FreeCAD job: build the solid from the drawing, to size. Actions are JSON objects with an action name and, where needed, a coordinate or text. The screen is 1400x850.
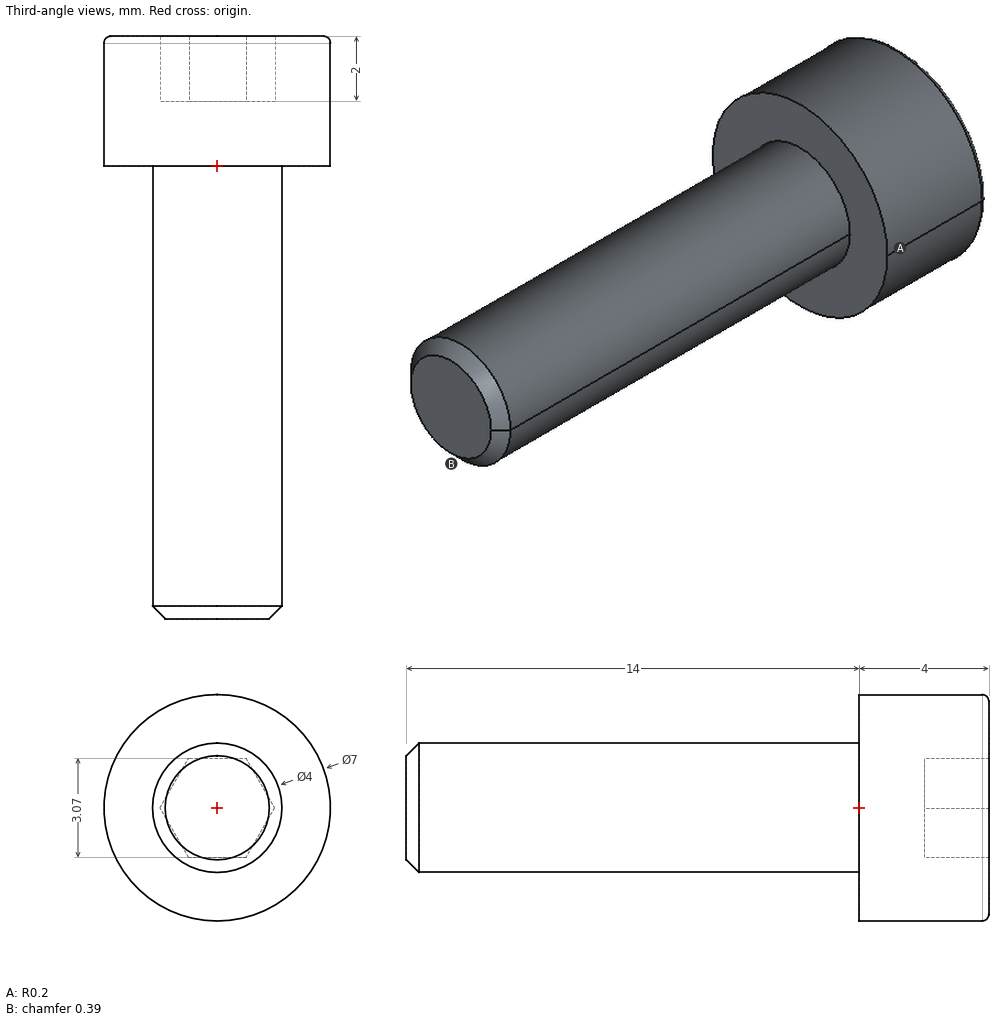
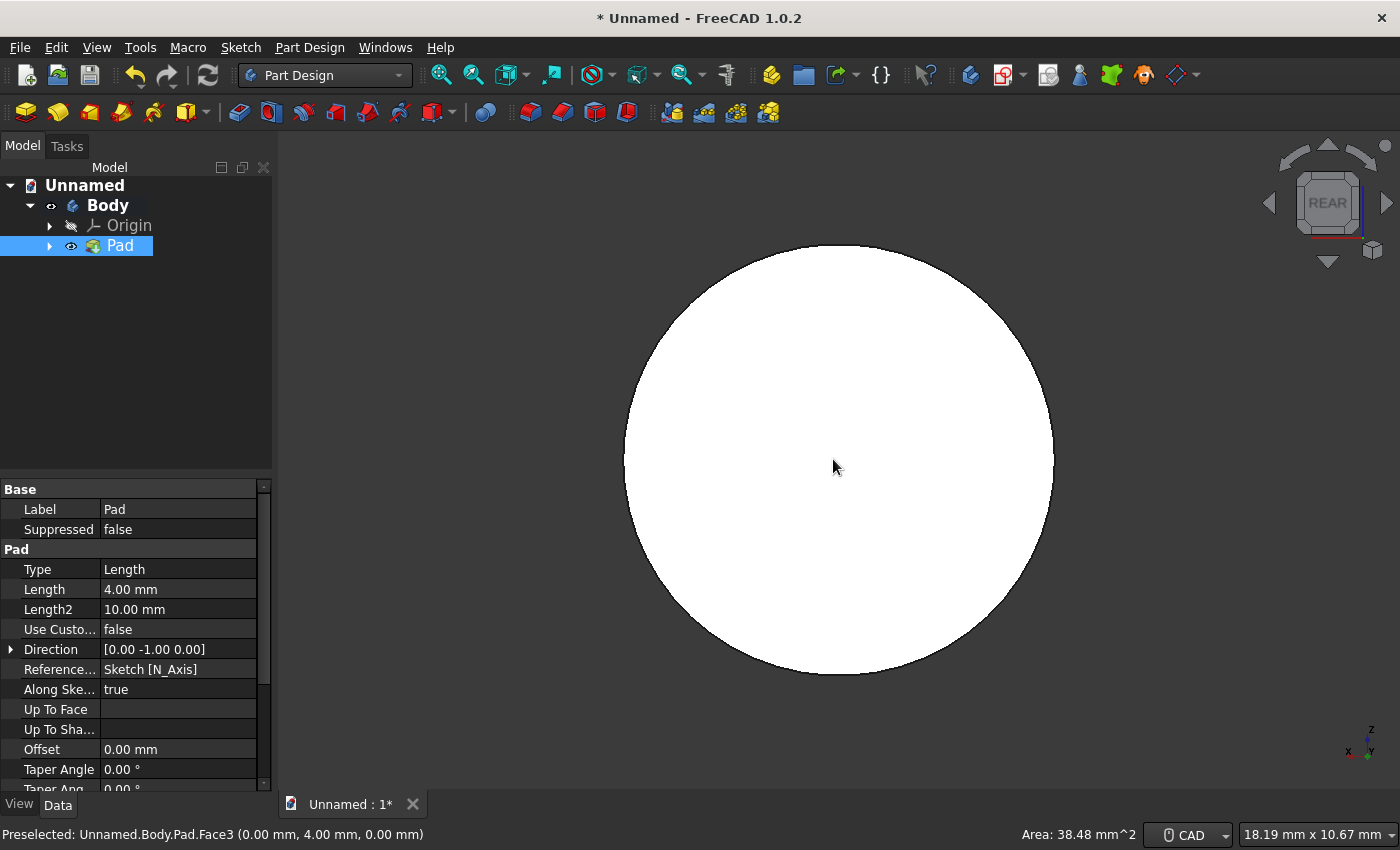
{"action": "left_click", "coordinate": [1004, 76]}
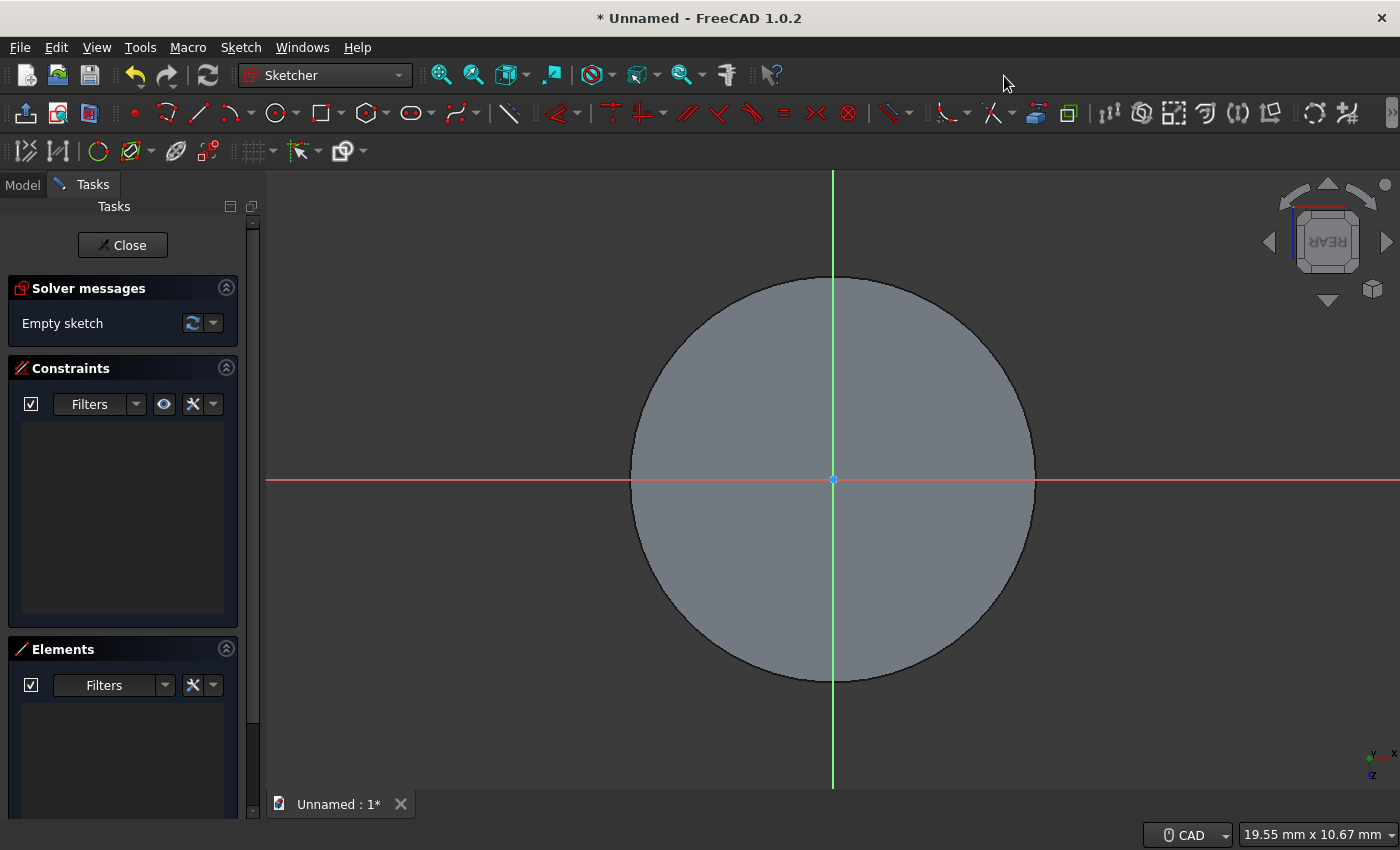
{"action": "scroll", "coordinate": [889, 480], "scroll_direction": "up", "scroll_amount": 4}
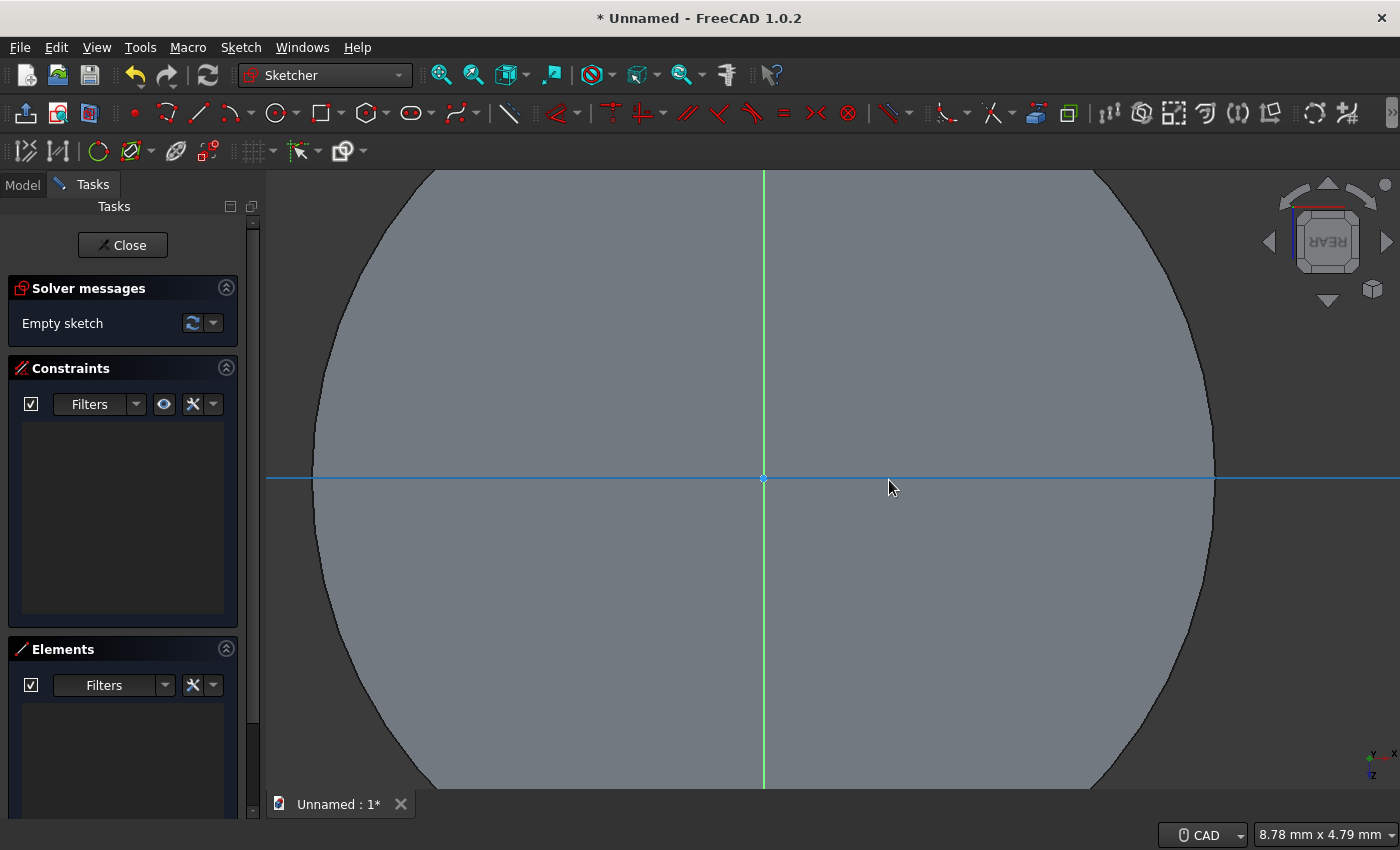
{"action": "left_click", "coordinate": [366, 114]}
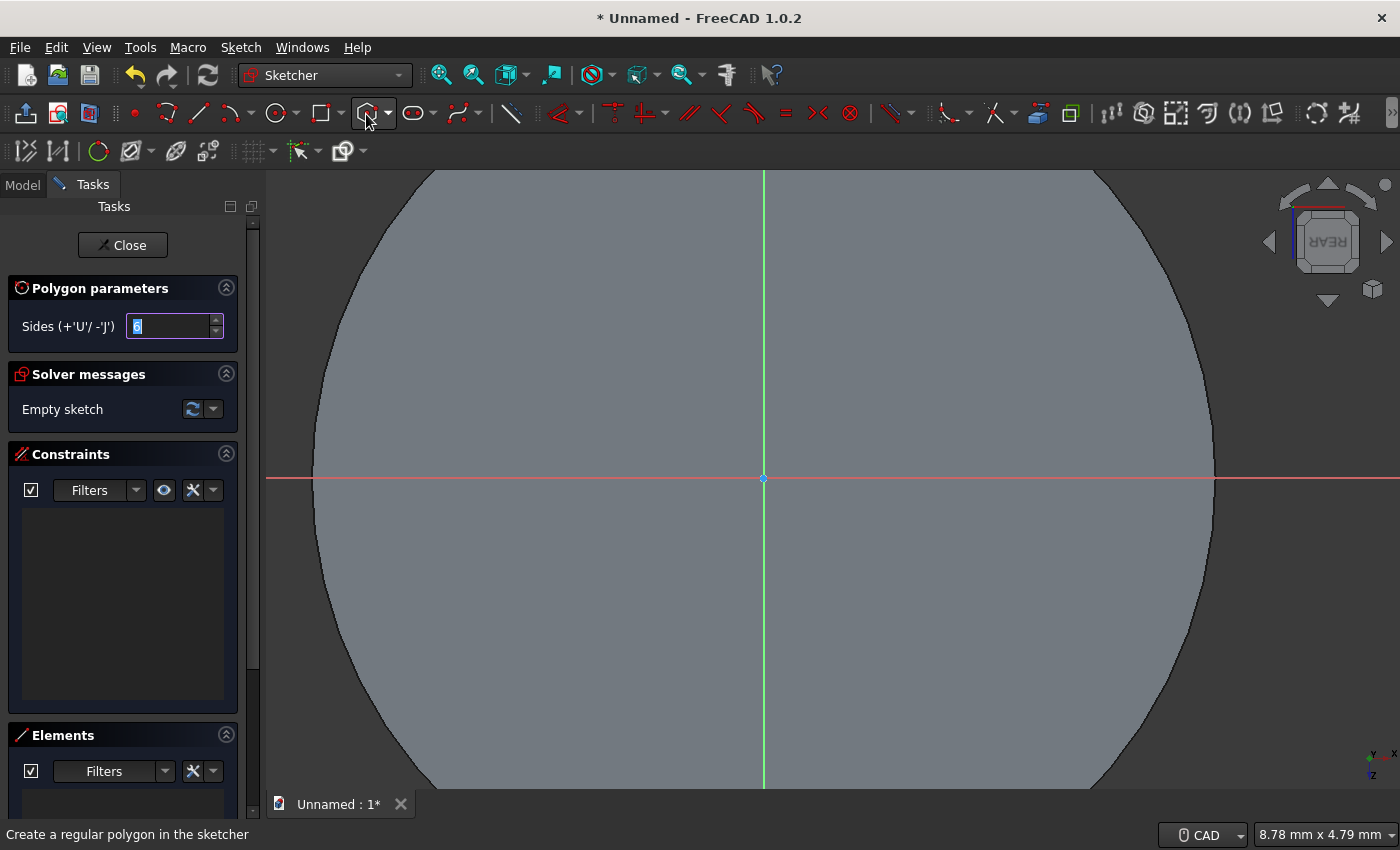
{"action": "left_click", "coordinate": [764, 478]}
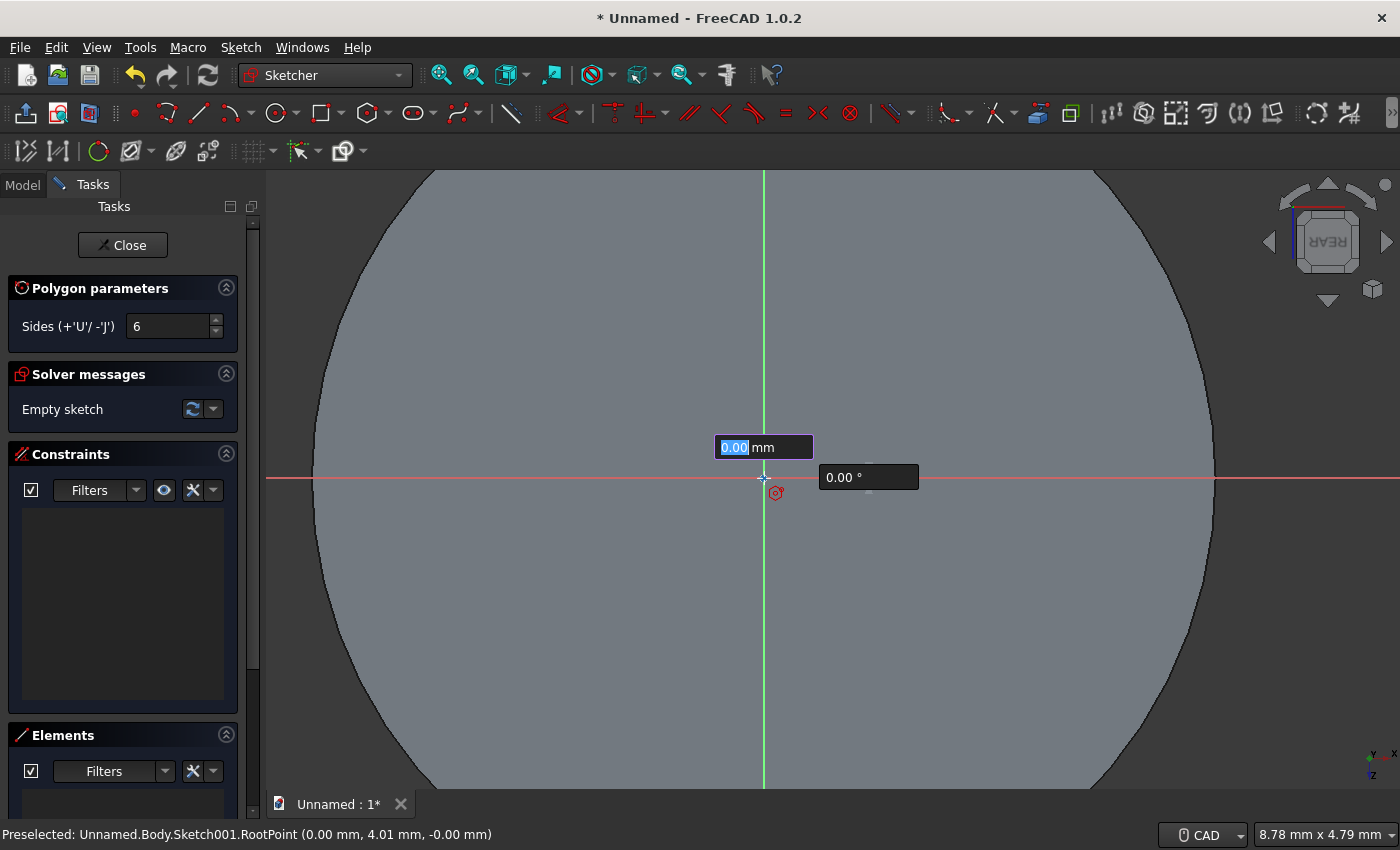
{"action": "left_click", "coordinate": [993, 478]}
{"action": "right_click", "coordinate": [993, 478]}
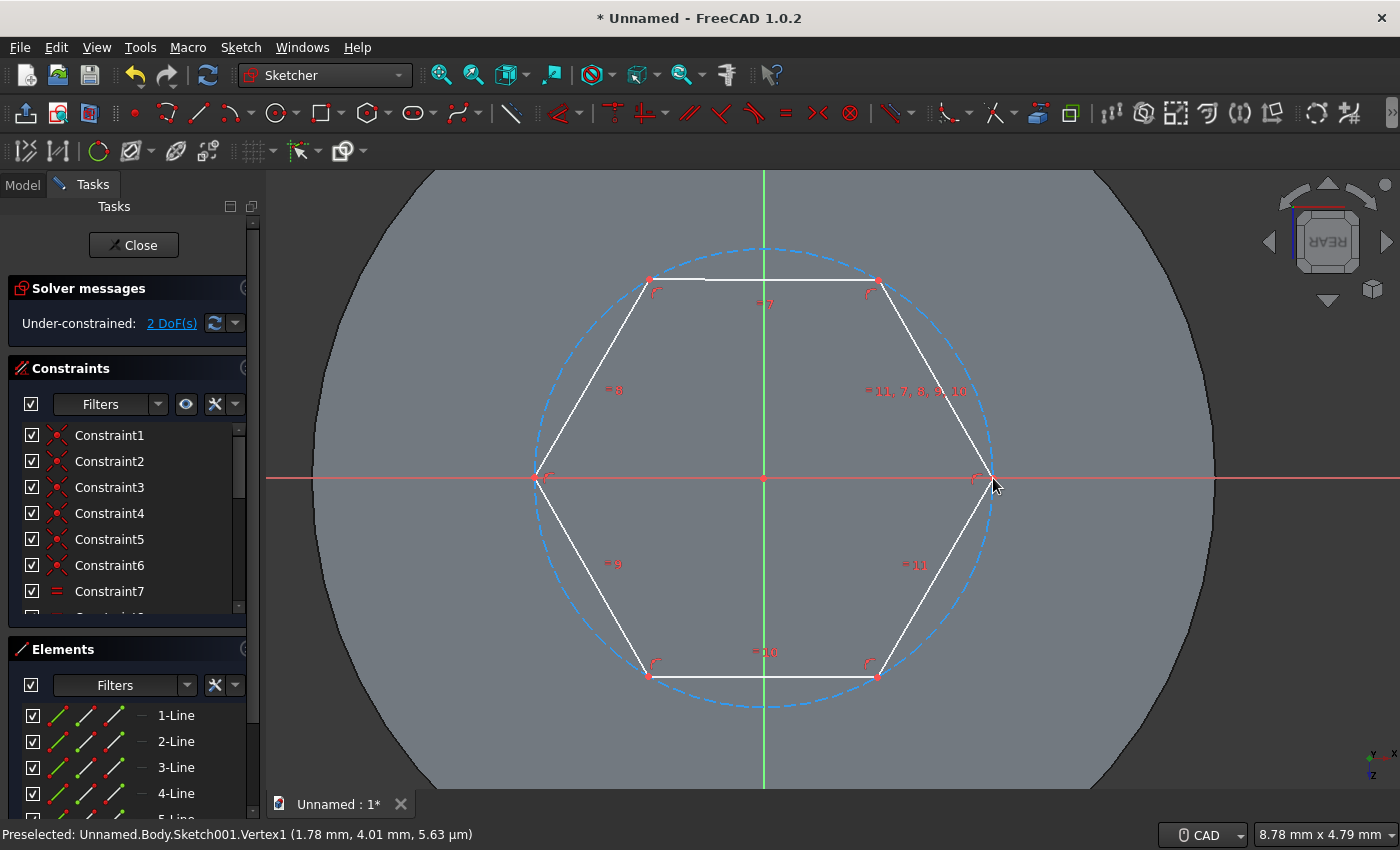
{"action": "left_click", "coordinate": [810, 280]}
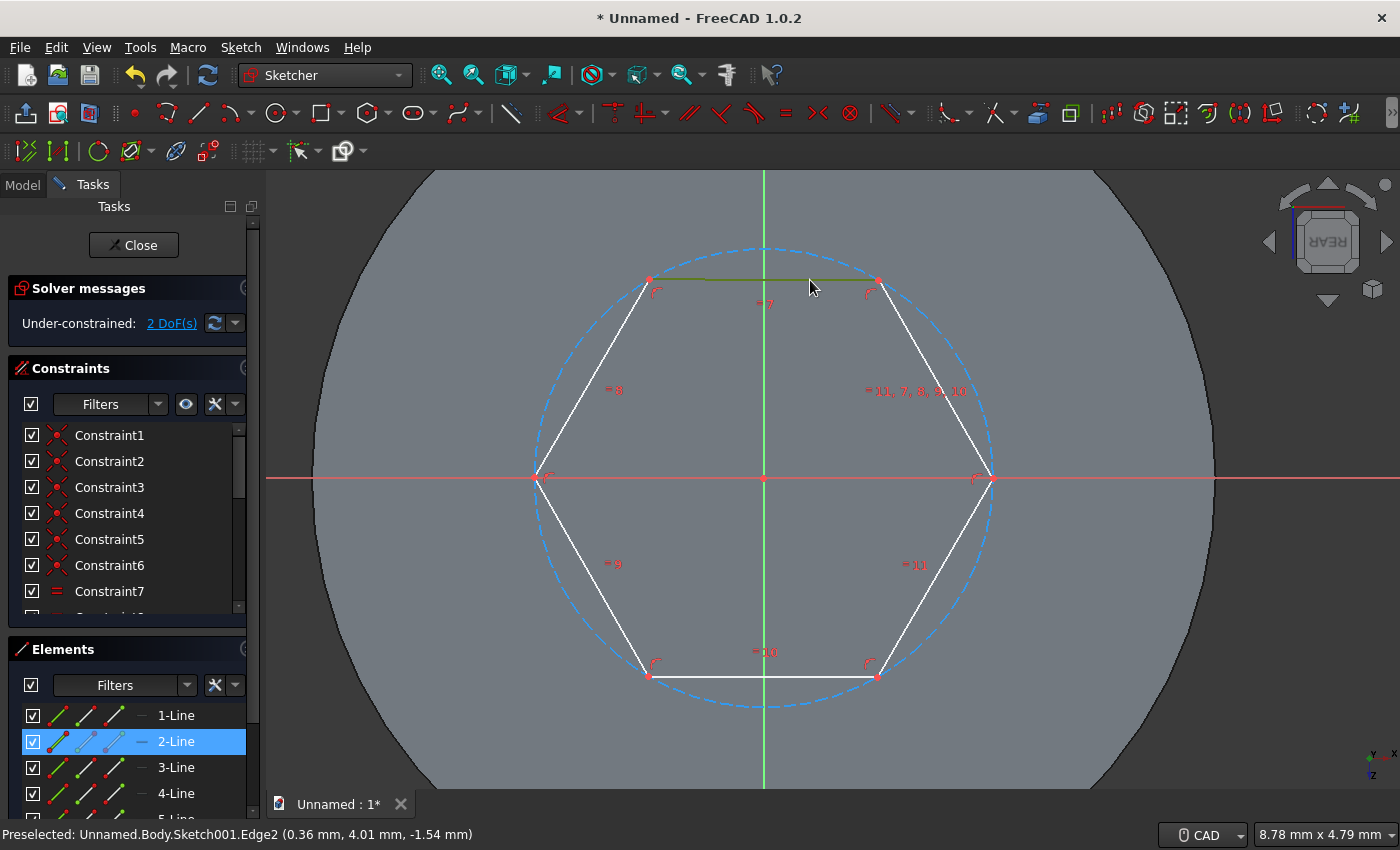
{"action": "left_click", "coordinate": [668, 114]}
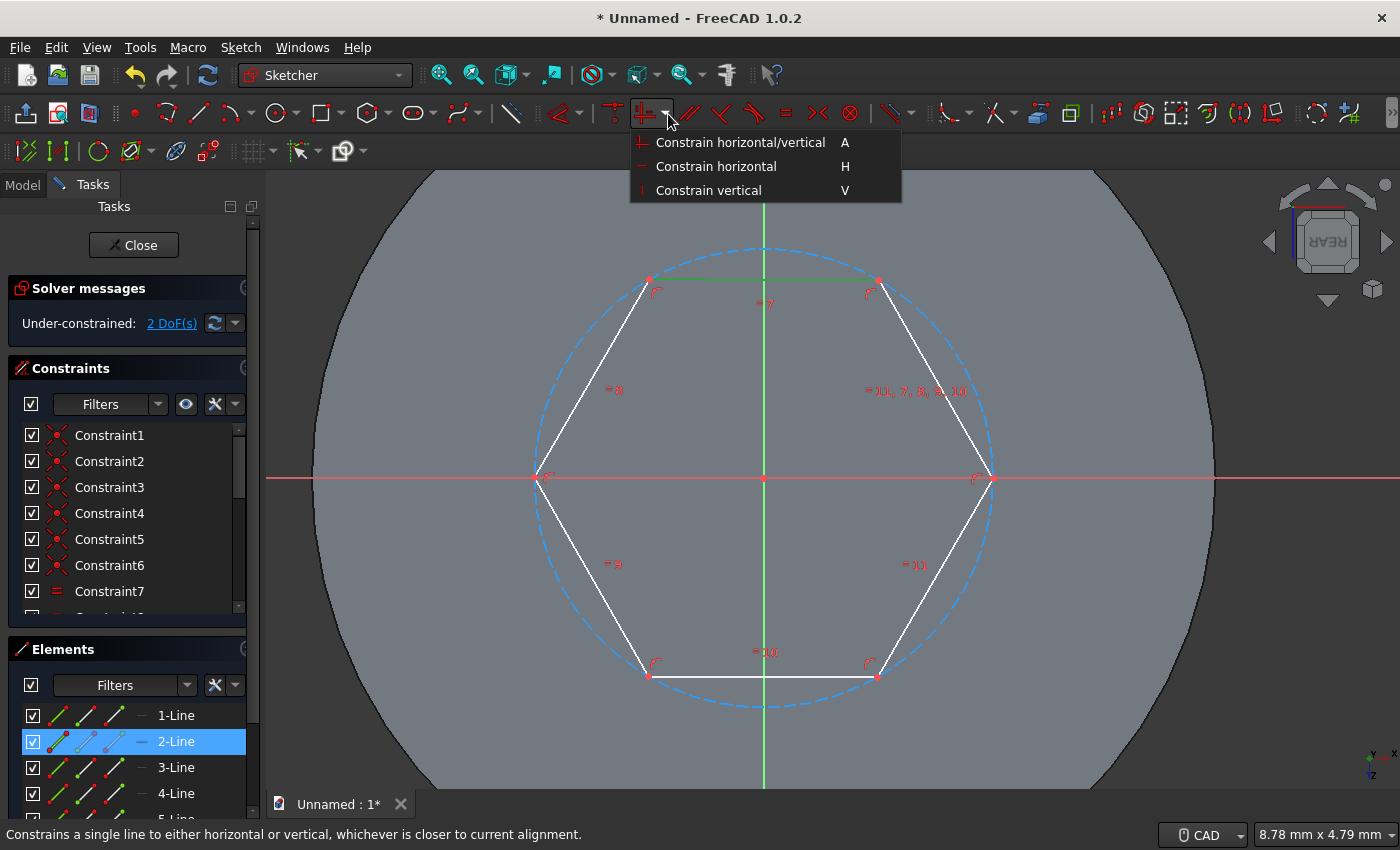
{"action": "left_click", "coordinate": [766, 166]}